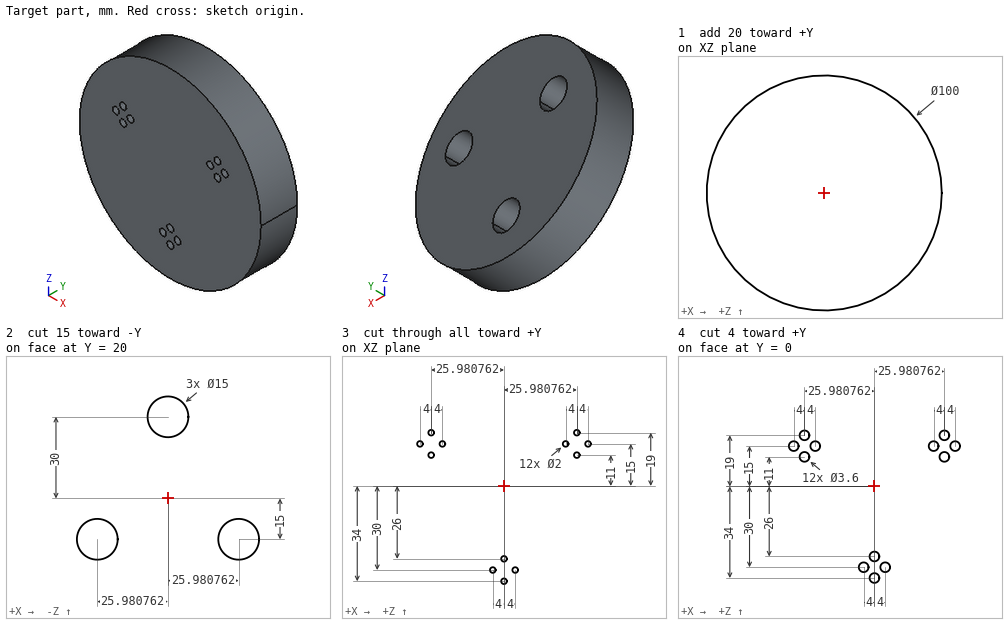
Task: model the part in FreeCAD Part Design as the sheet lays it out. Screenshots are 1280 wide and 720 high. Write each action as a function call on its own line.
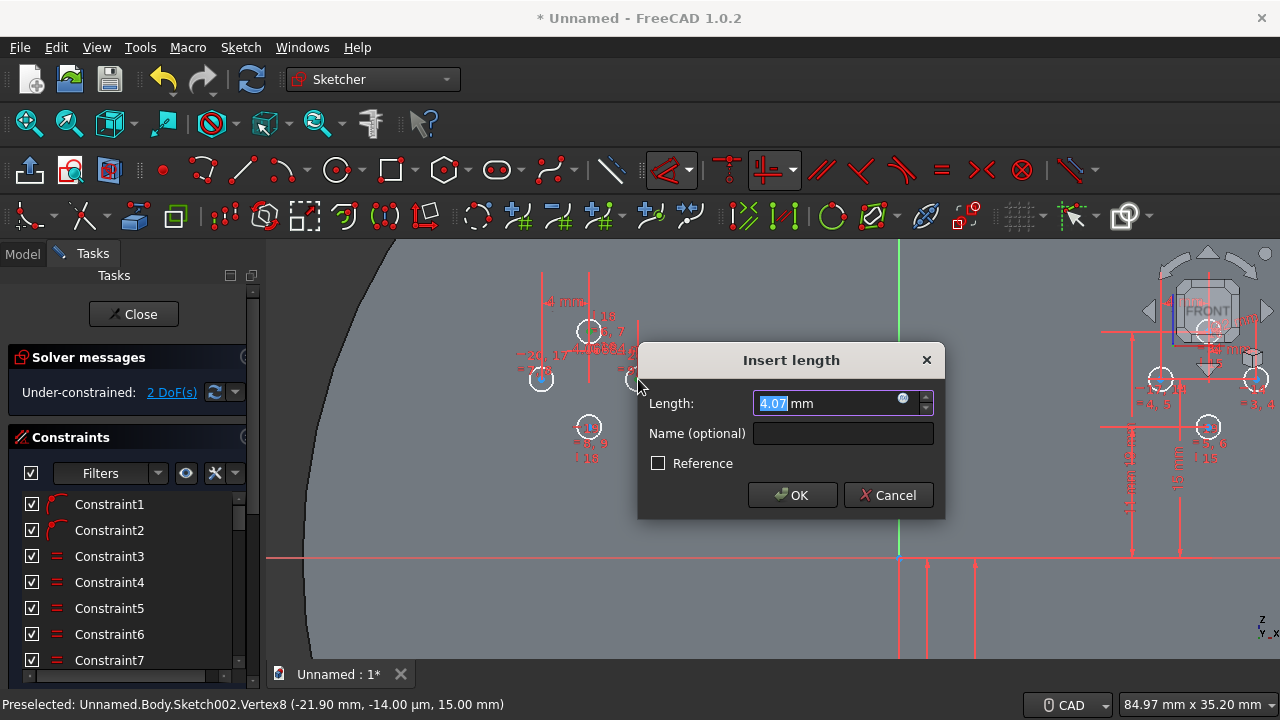
text(4)
key(Return)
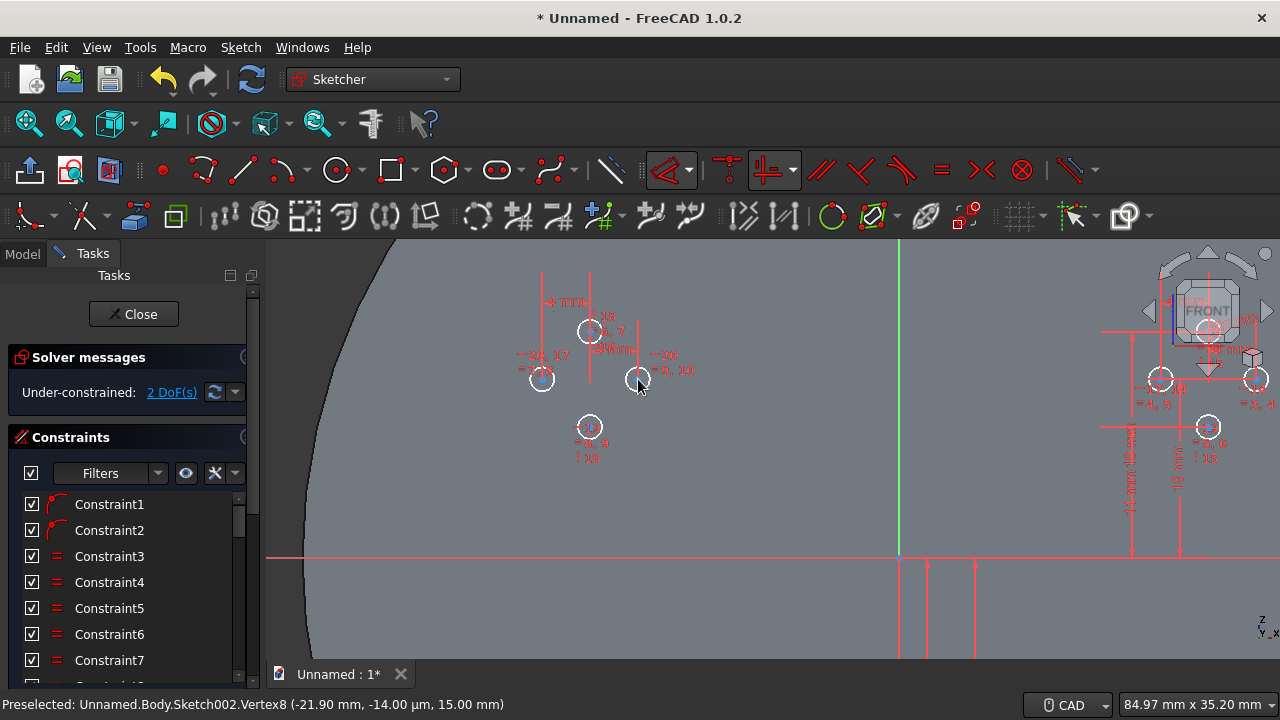
scroll(591, 333, down, 5)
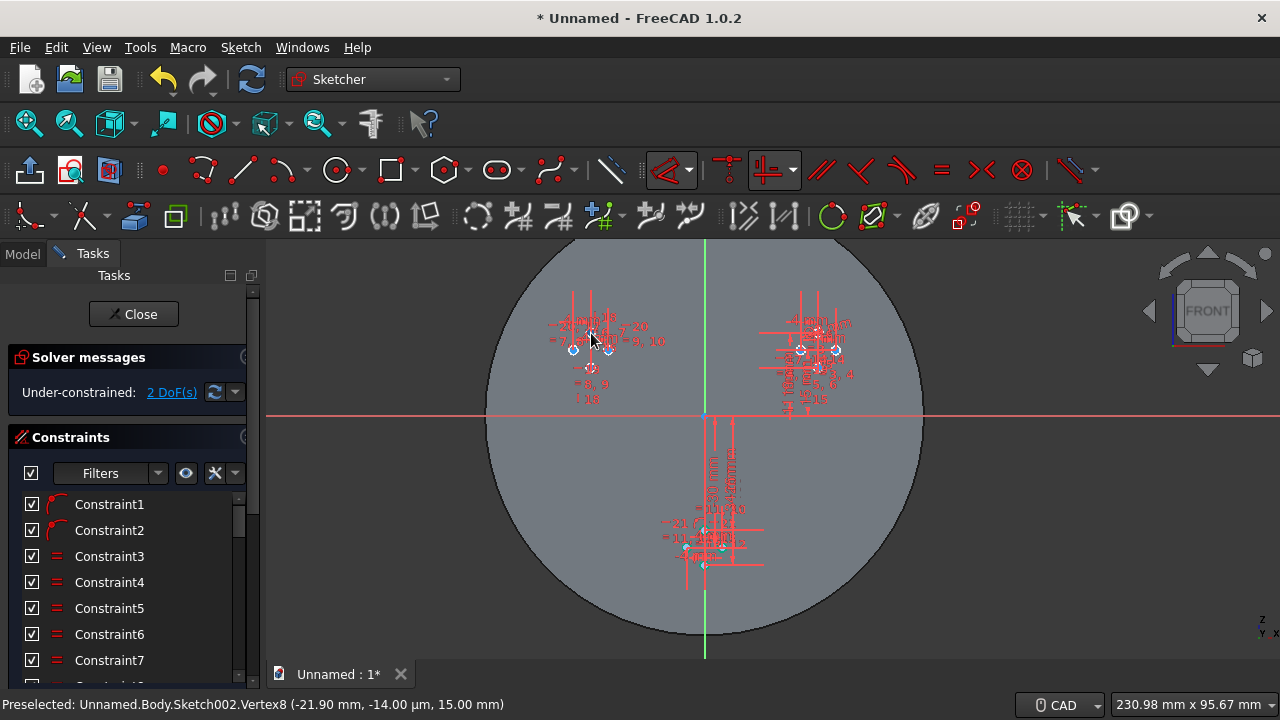
click(818, 333)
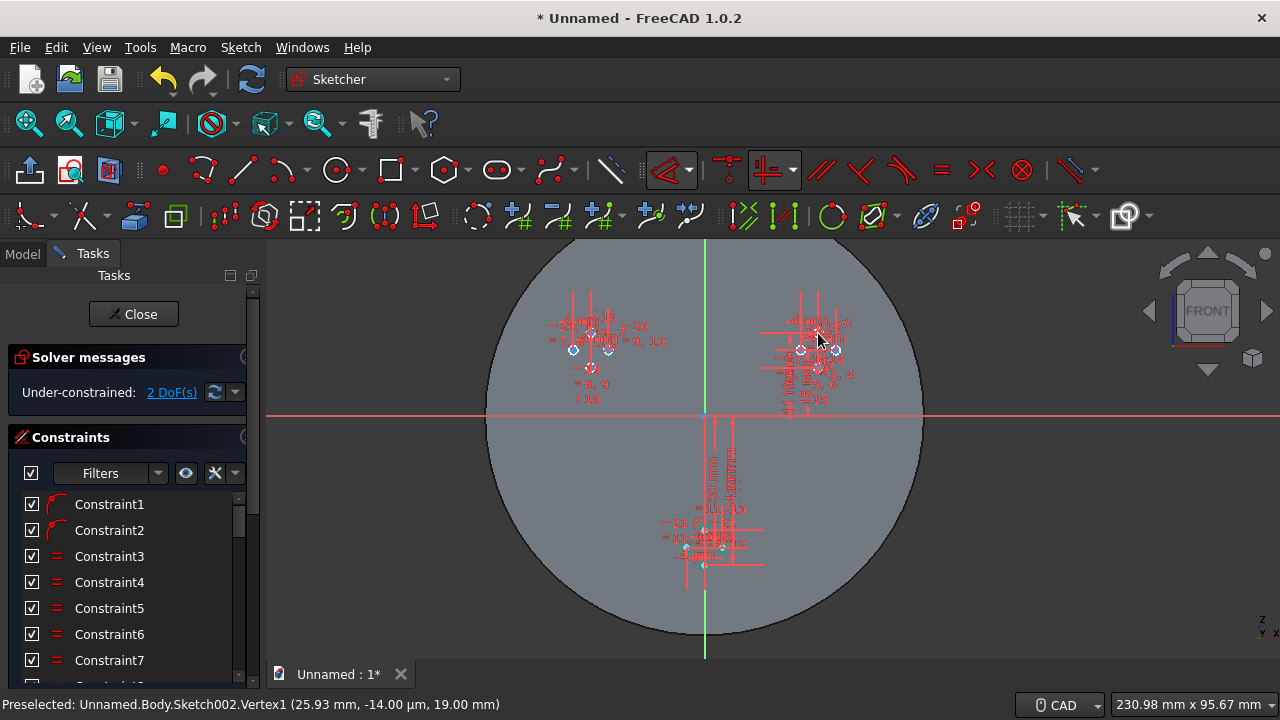
click(692, 170)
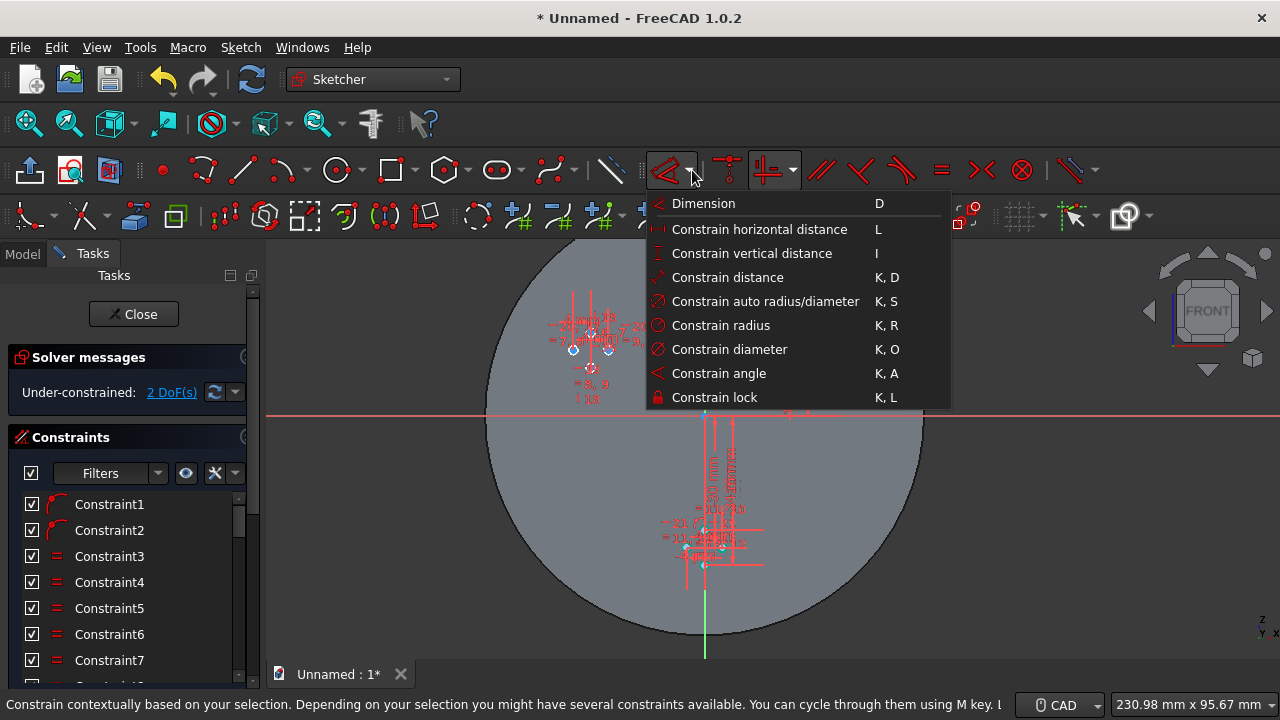
click(799, 229)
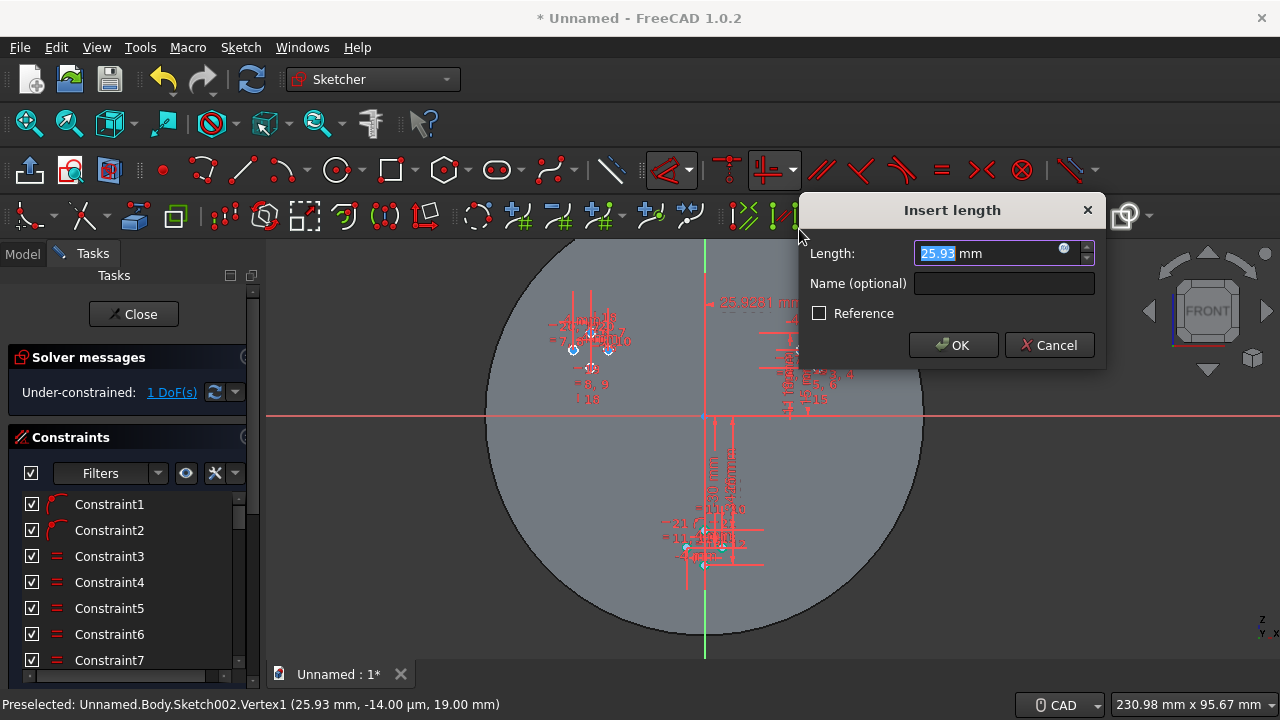
text(25.980762)
key(Return)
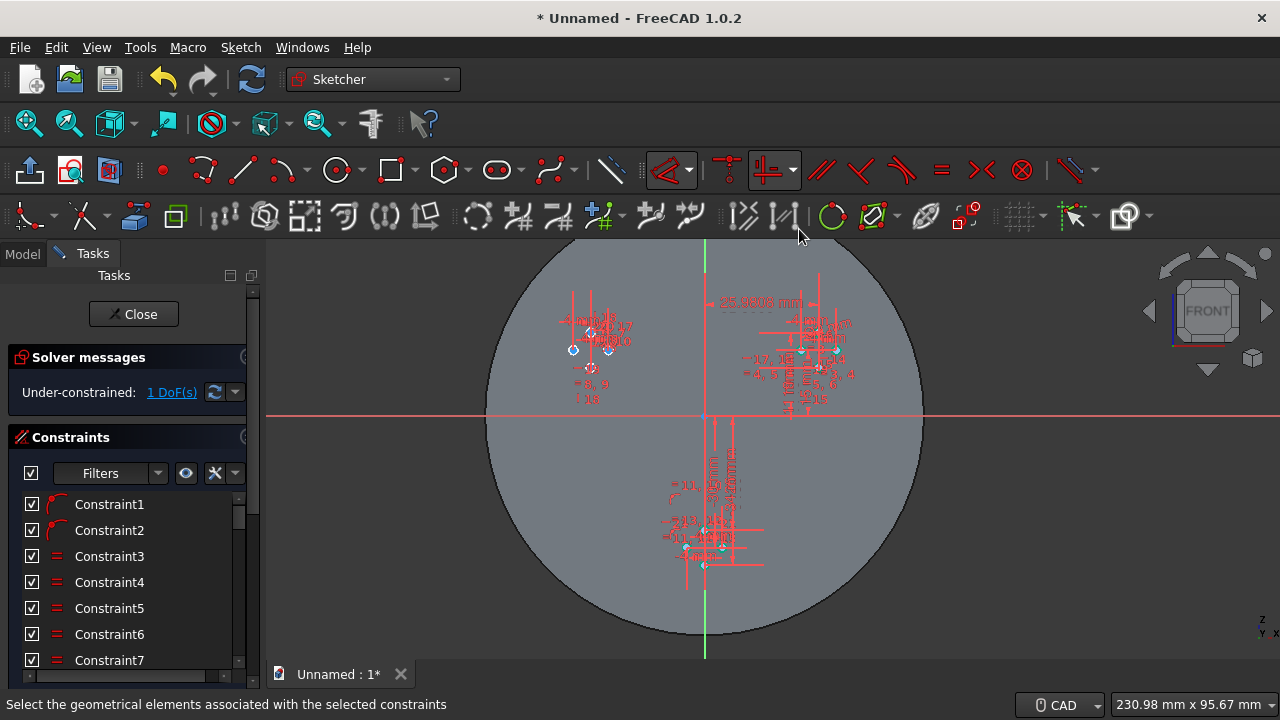
scroll(591, 333, up, 4)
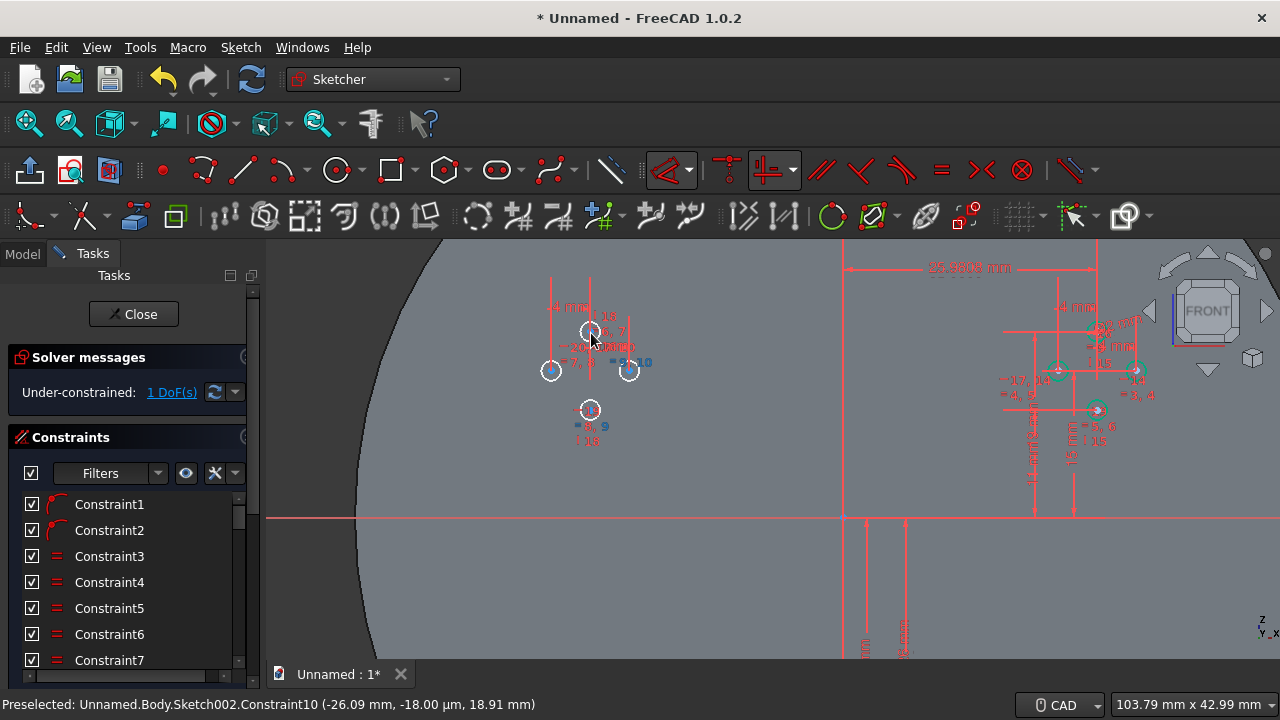
click(590, 332)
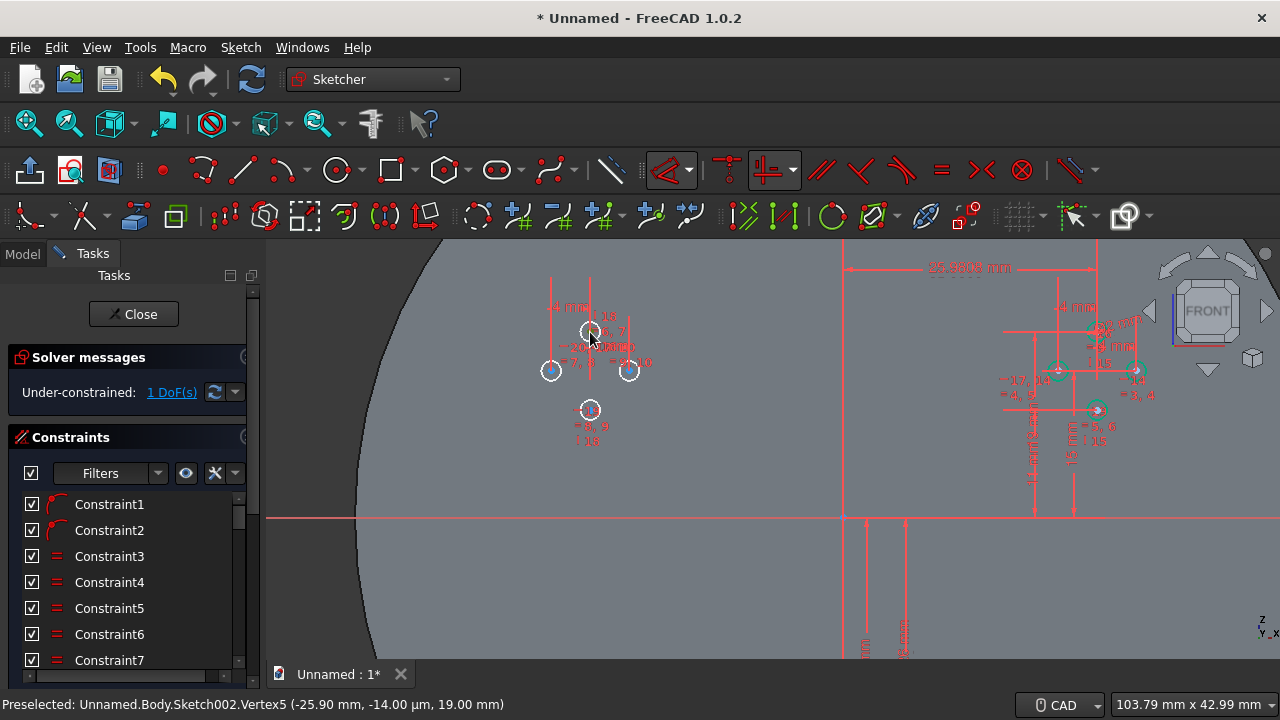
click(692, 170)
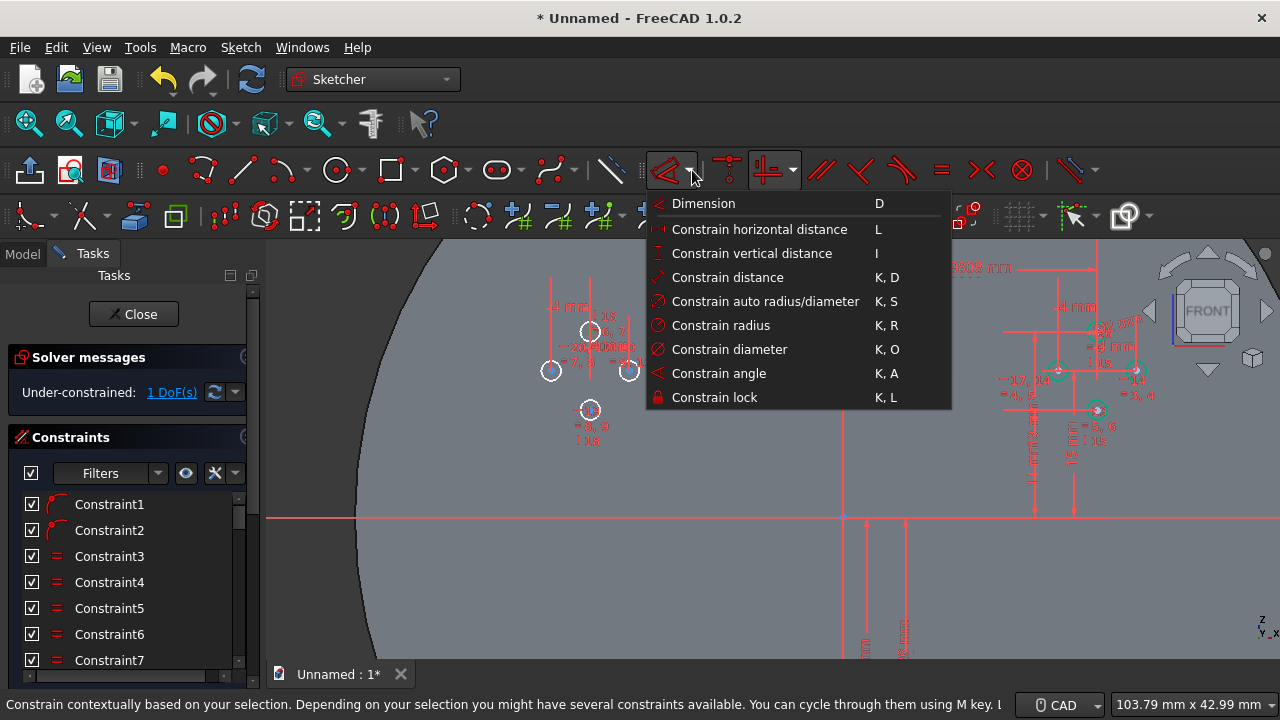
click(799, 229)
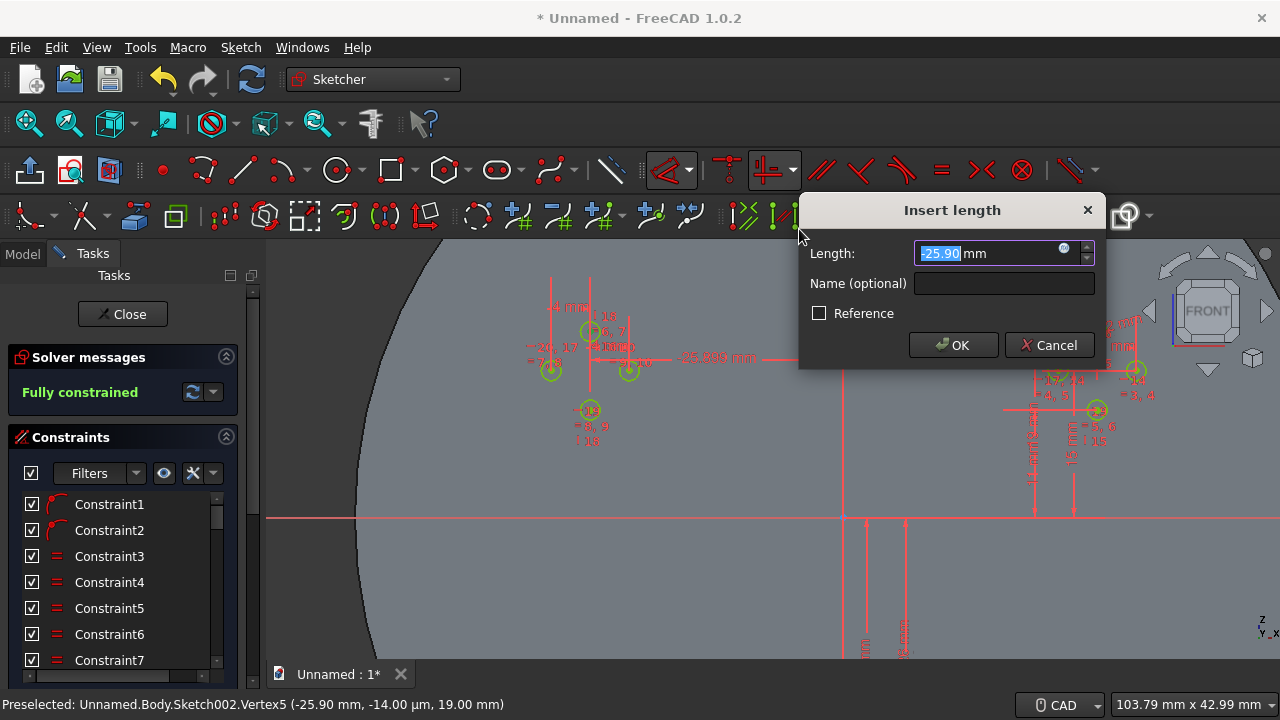
text(-25.980762)
key(Return)